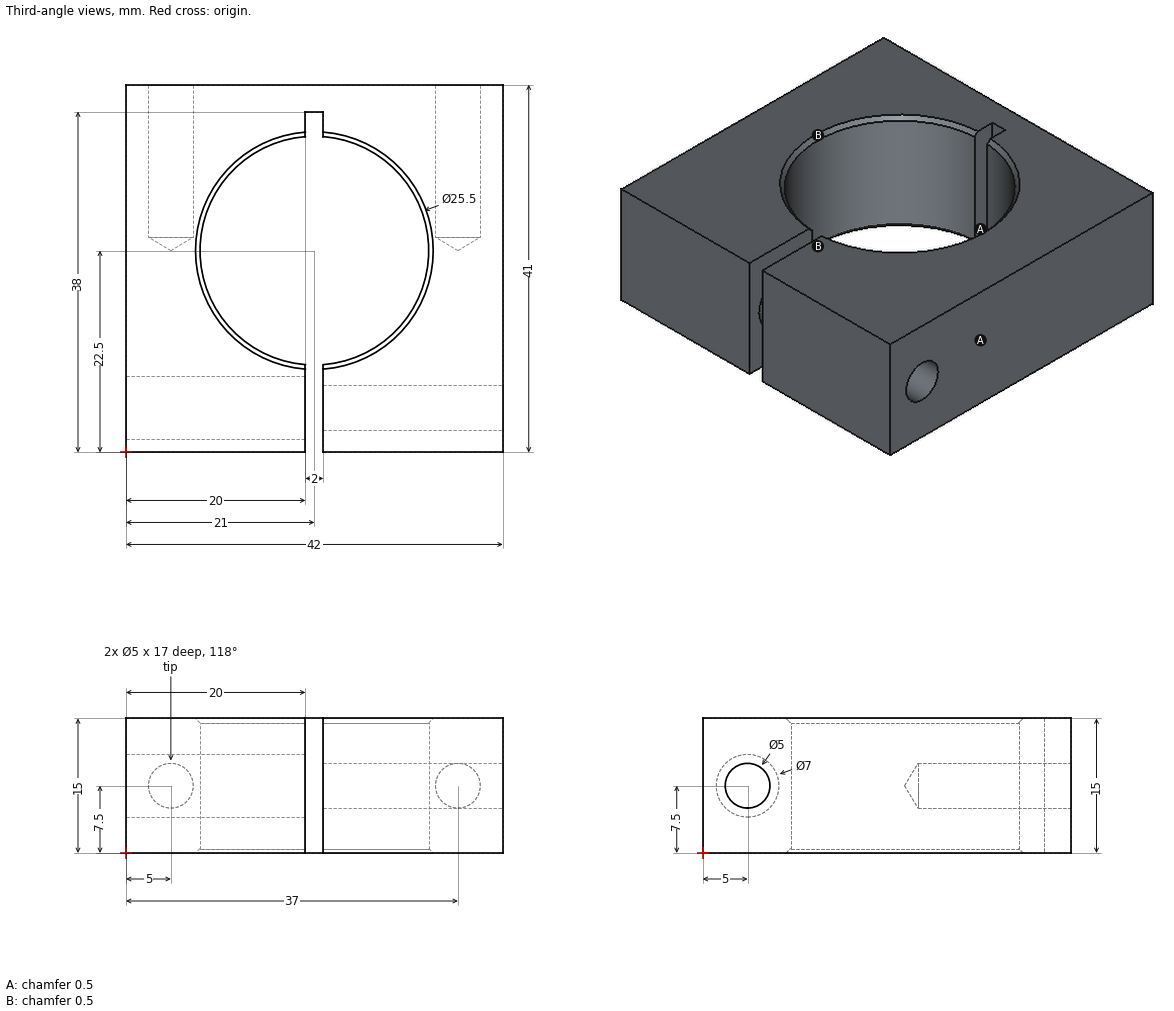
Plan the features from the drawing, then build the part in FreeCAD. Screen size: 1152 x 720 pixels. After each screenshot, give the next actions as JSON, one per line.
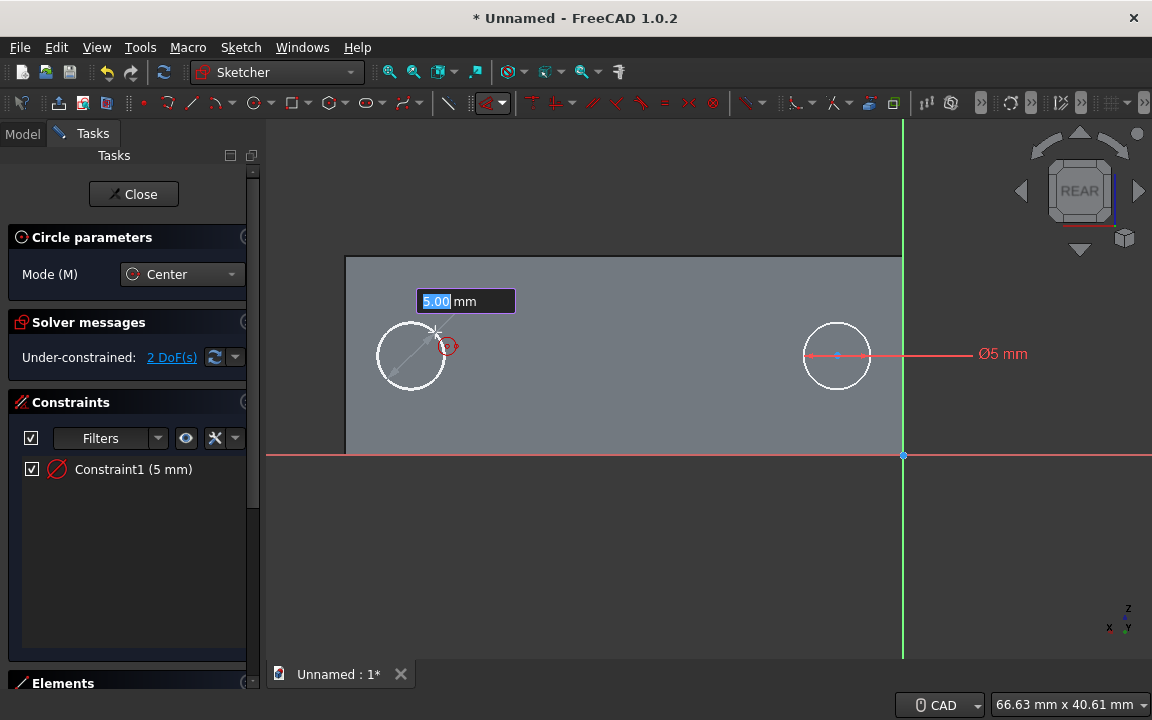
{"action": "type", "text": "5"}
{"action": "key", "text": "Return"}
{"action": "key", "text": "Escape"}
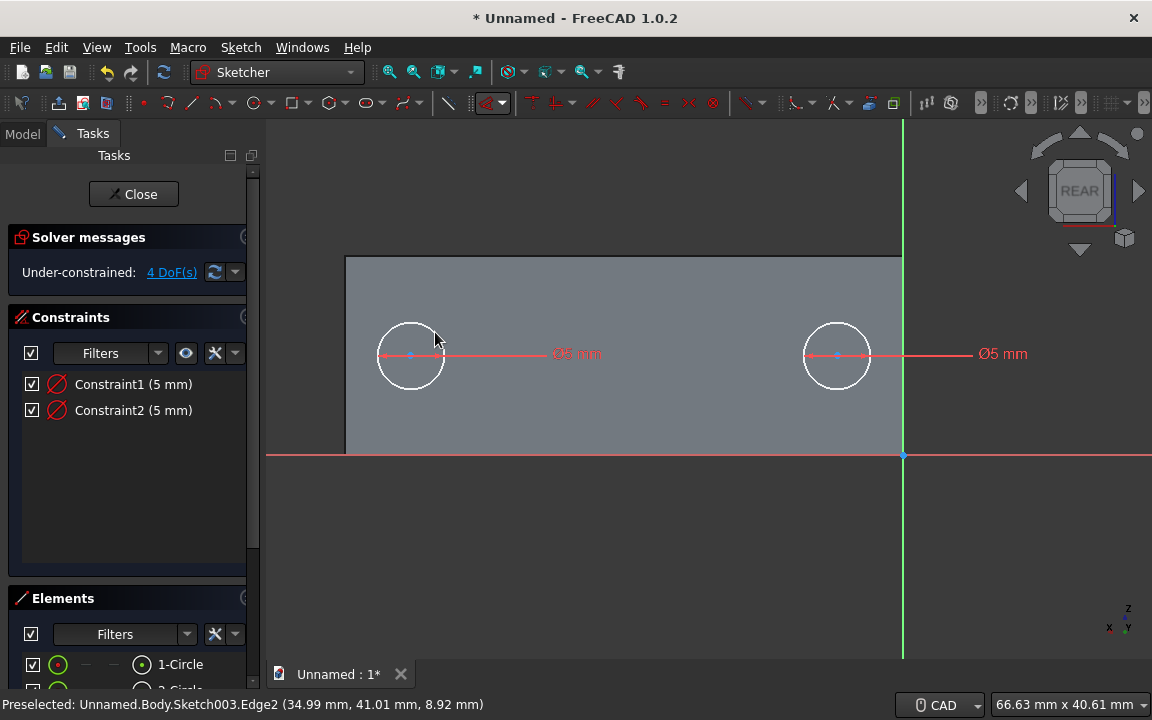
{"action": "left_click", "coordinate": [837, 356]}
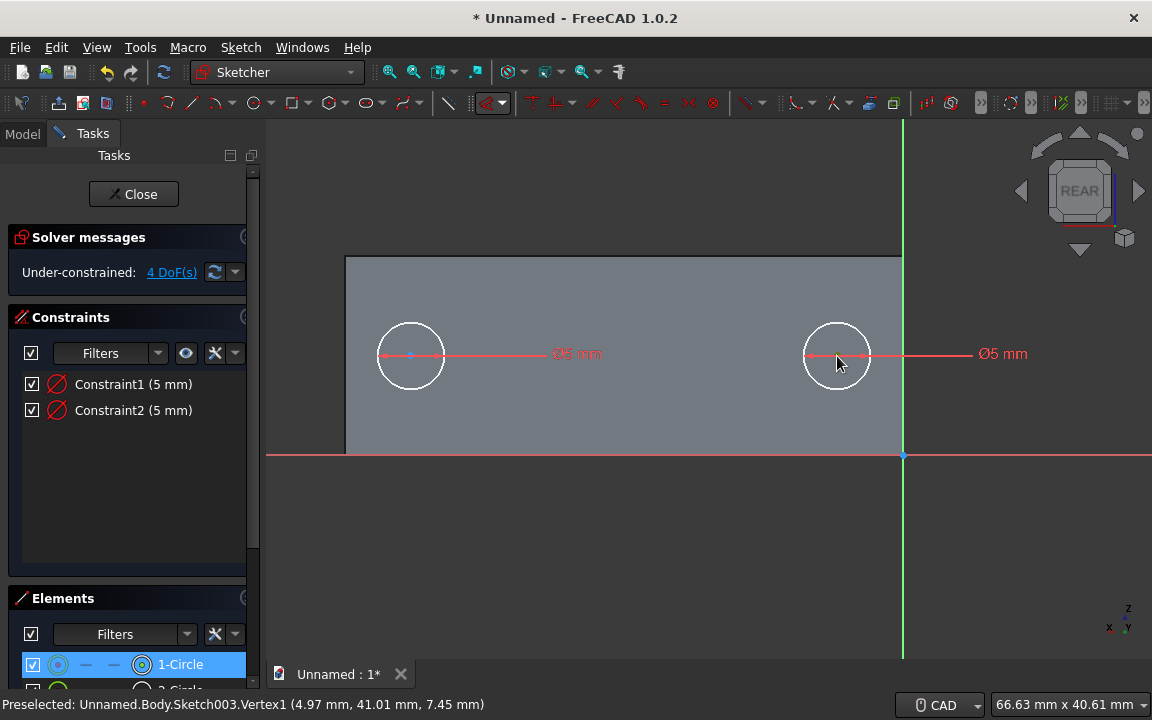
{"action": "left_click", "coordinate": [411, 356]}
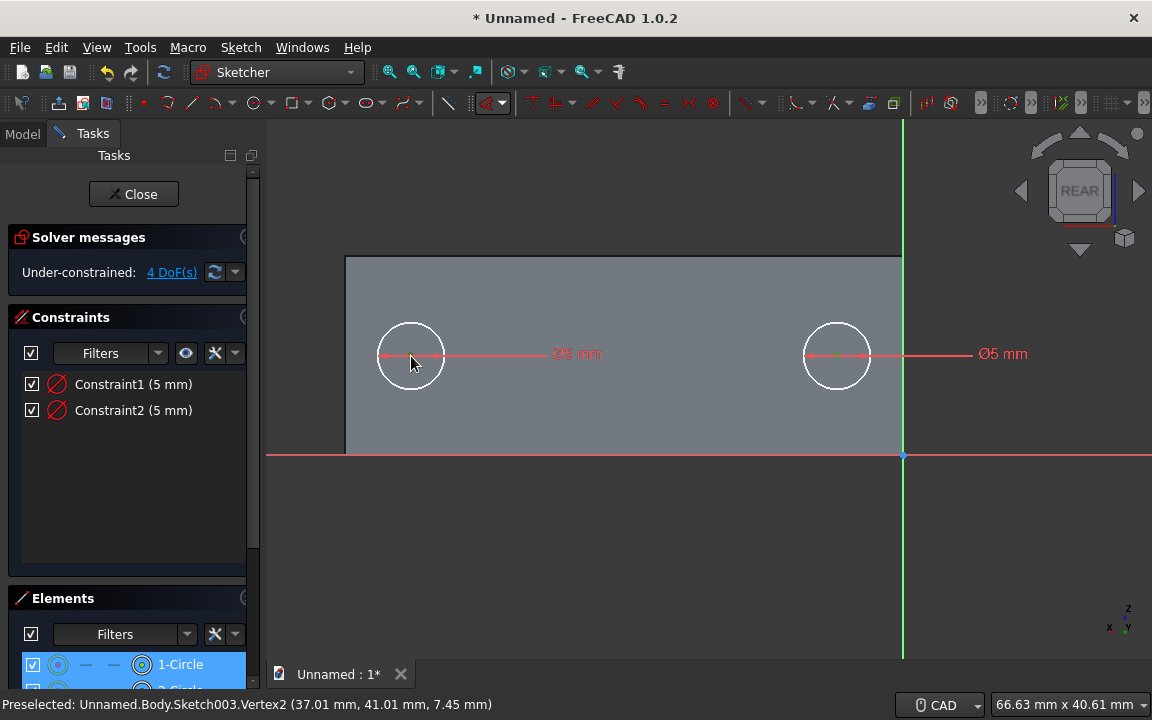
{"action": "left_click", "coordinate": [574, 104]}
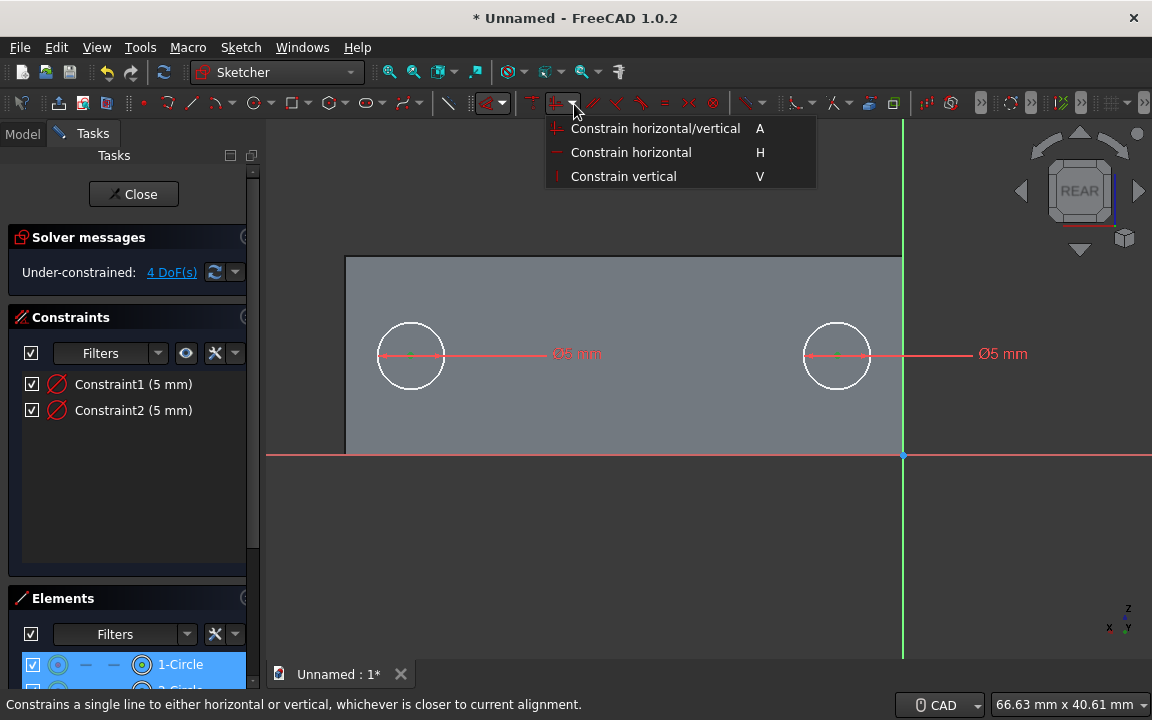
{"action": "left_click", "coordinate": [681, 152]}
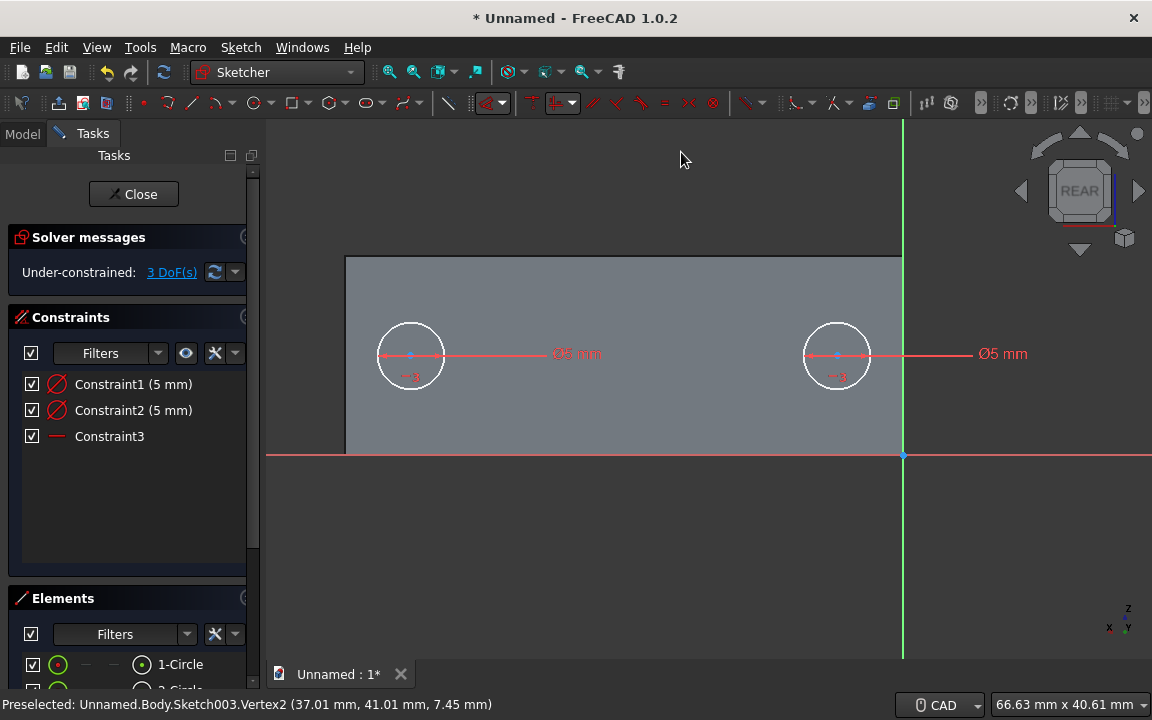
{"action": "left_click", "coordinate": [837, 356]}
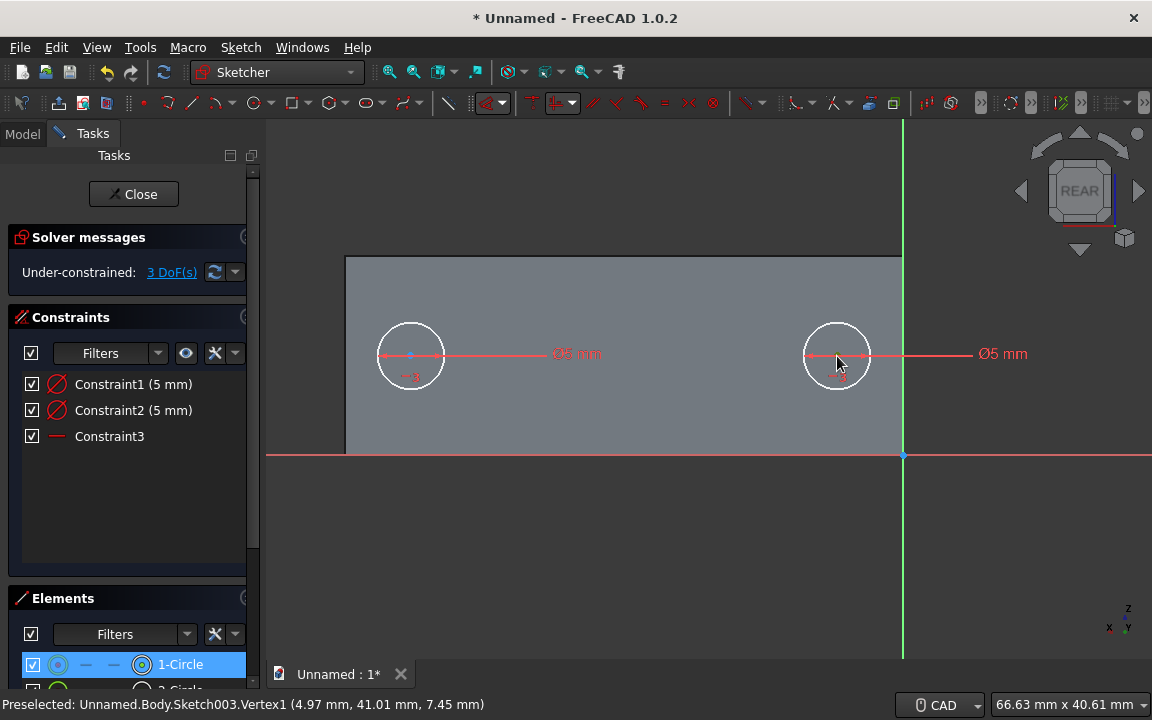
{"action": "left_click", "coordinate": [504, 104]}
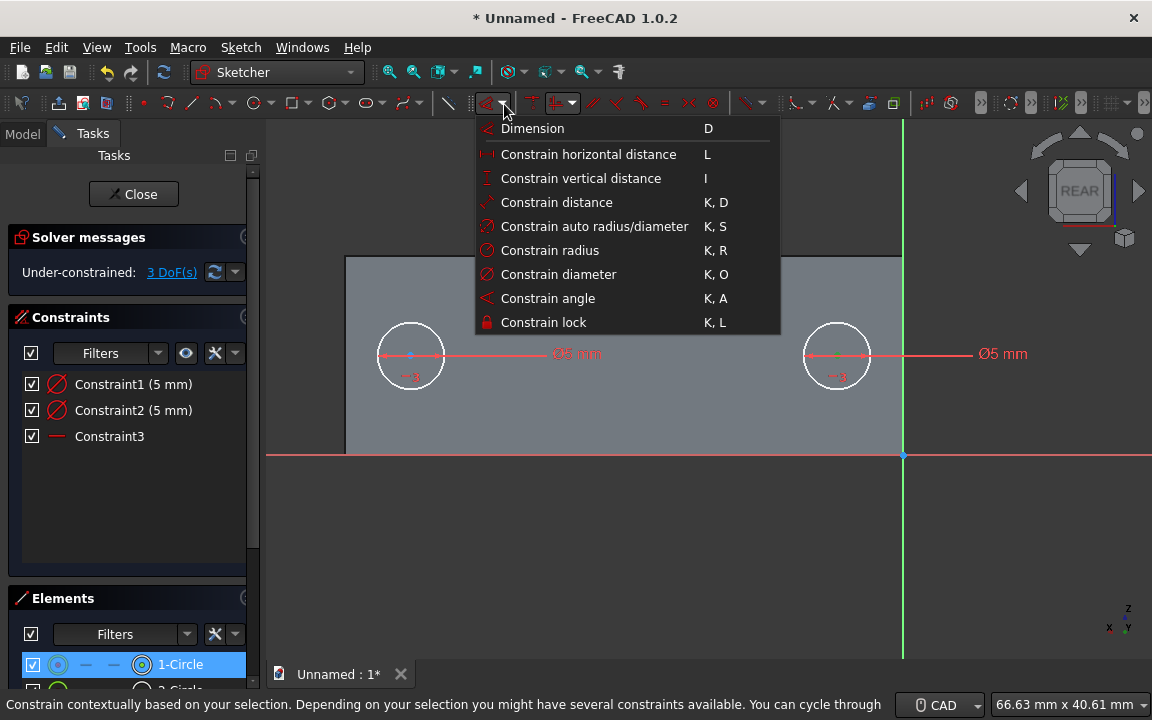
{"action": "left_click", "coordinate": [628, 154]}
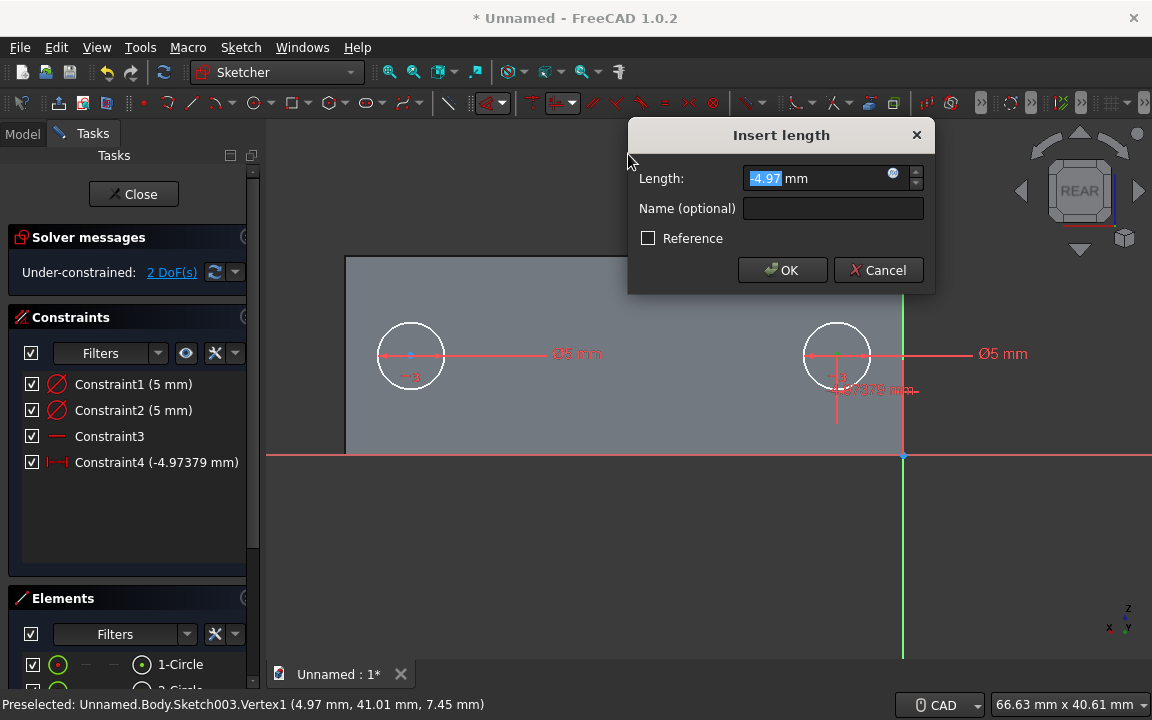
{"action": "type", "text": "-5"}
{"action": "key", "text": "Return"}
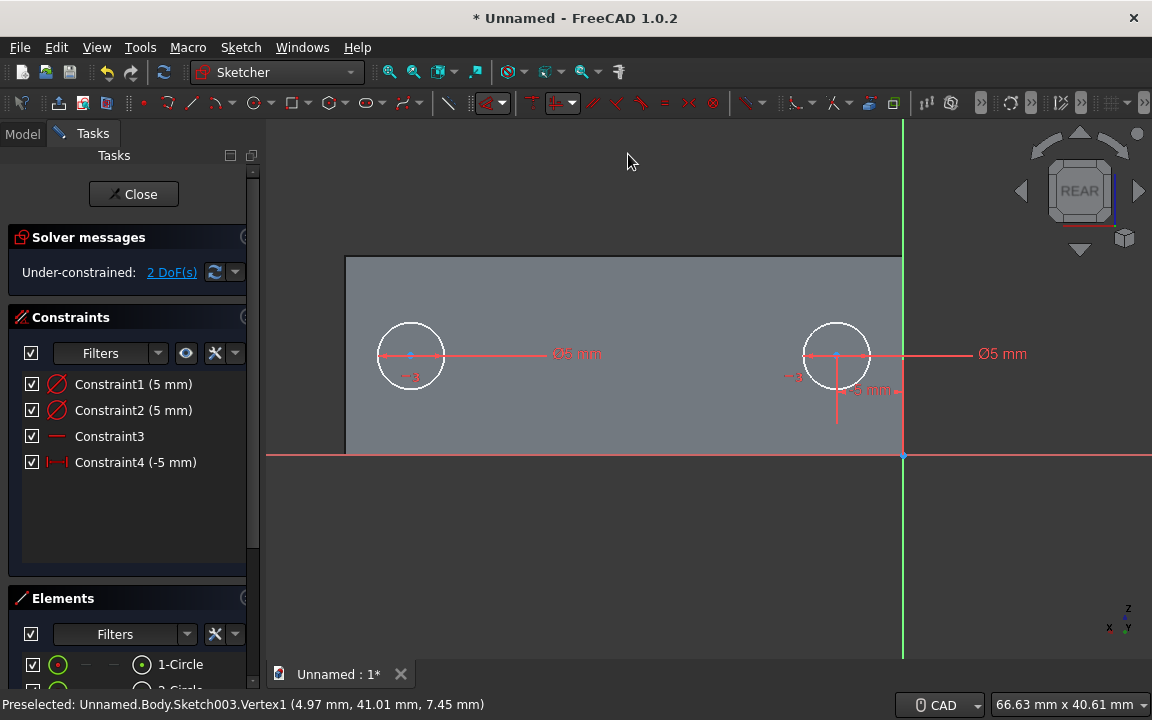
{"action": "left_click", "coordinate": [411, 356]}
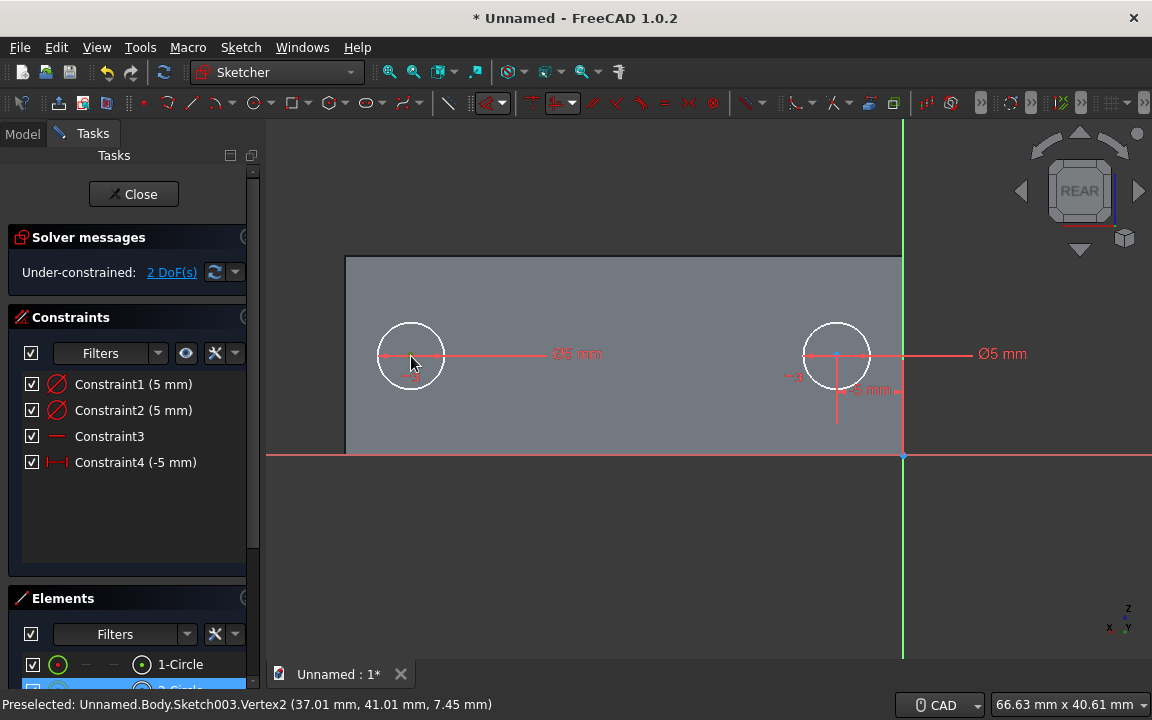
{"action": "left_click", "coordinate": [504, 104]}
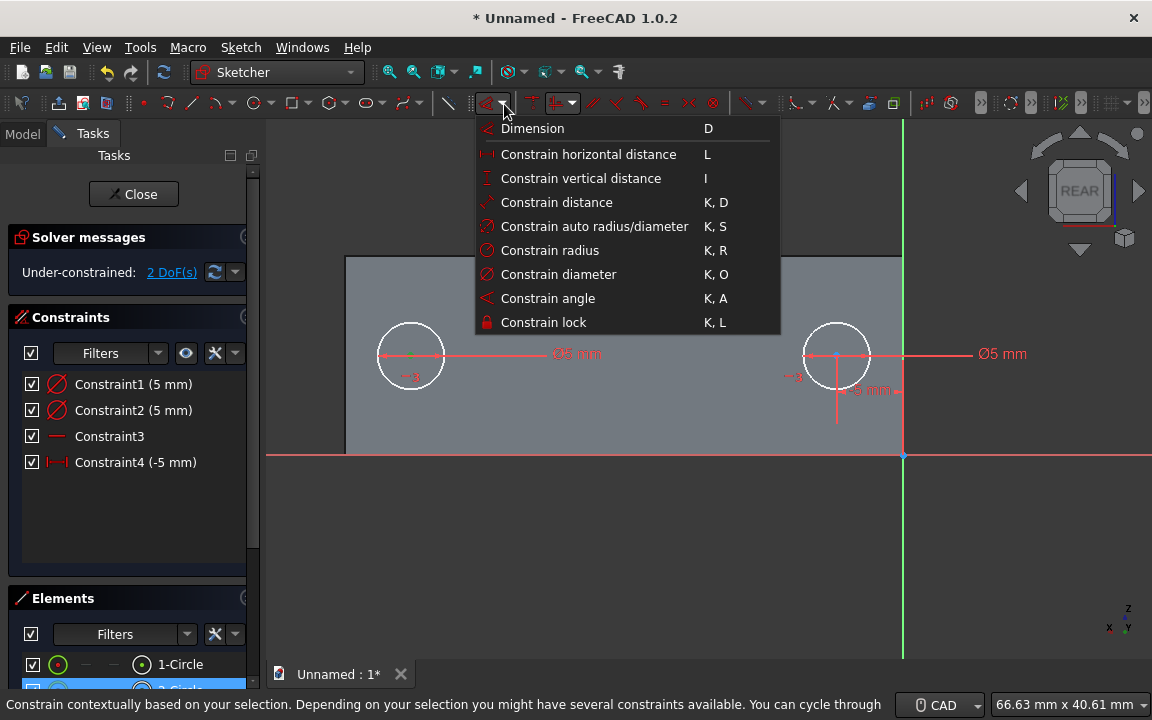
{"action": "left_click", "coordinate": [628, 154]}